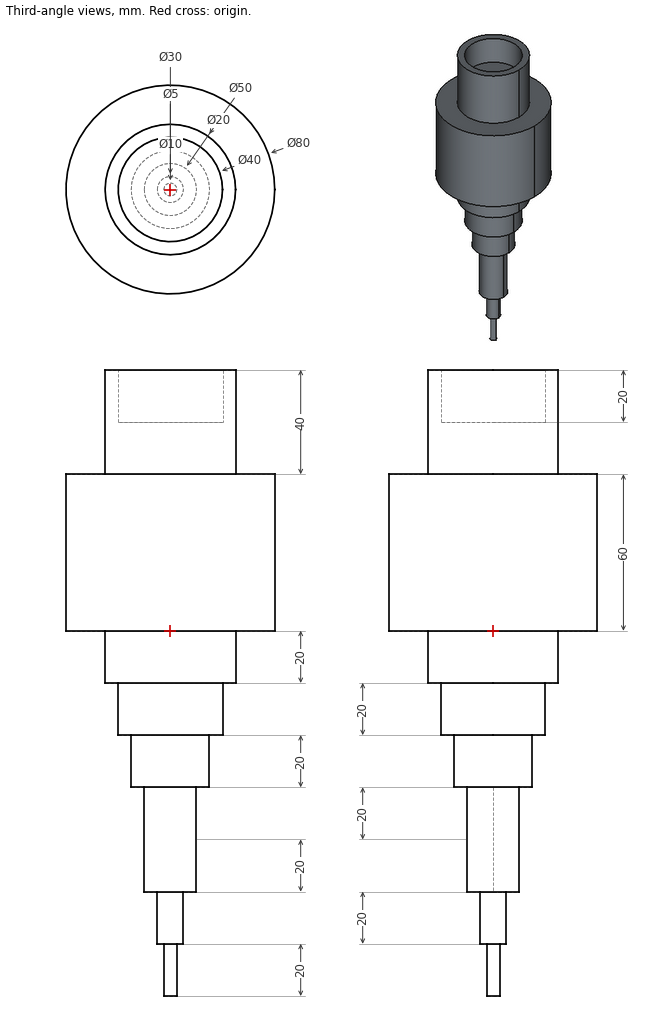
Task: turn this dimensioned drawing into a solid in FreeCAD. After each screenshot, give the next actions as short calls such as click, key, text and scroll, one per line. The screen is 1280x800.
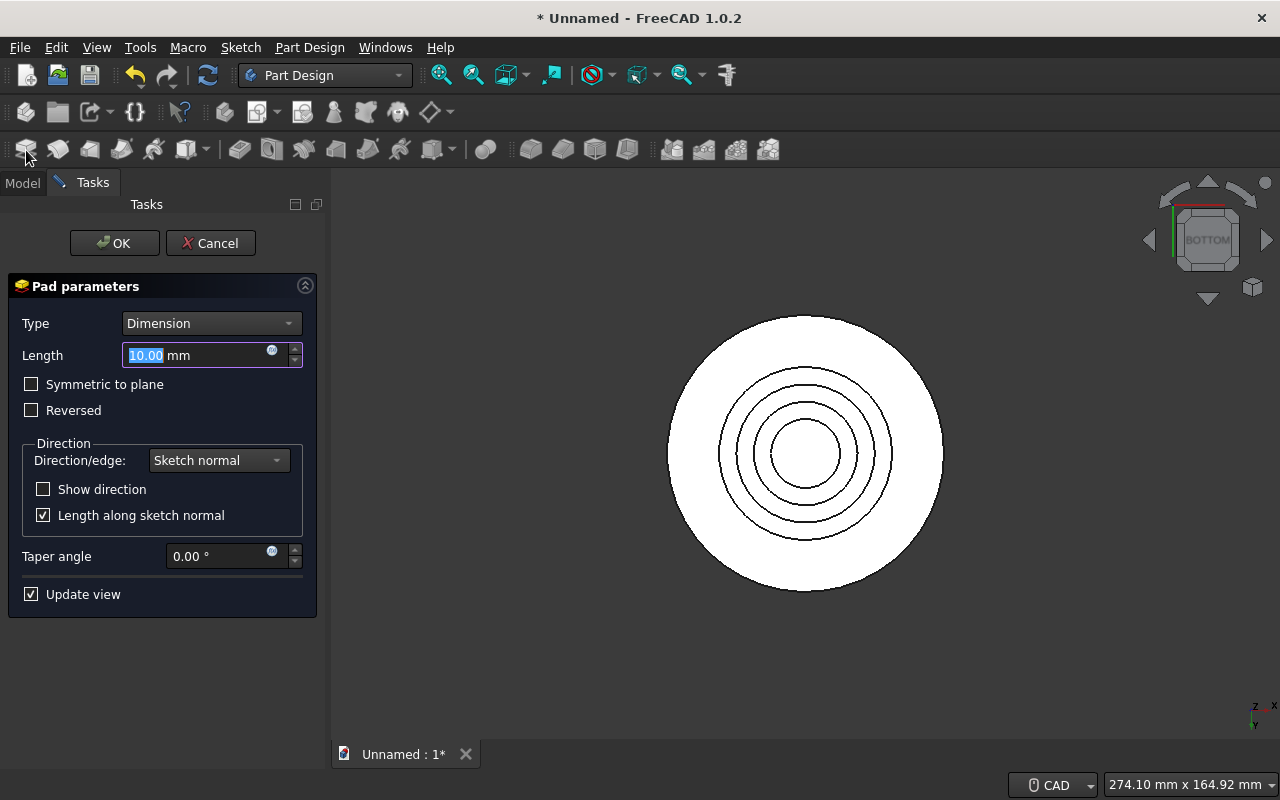
text(20)
key(Tab)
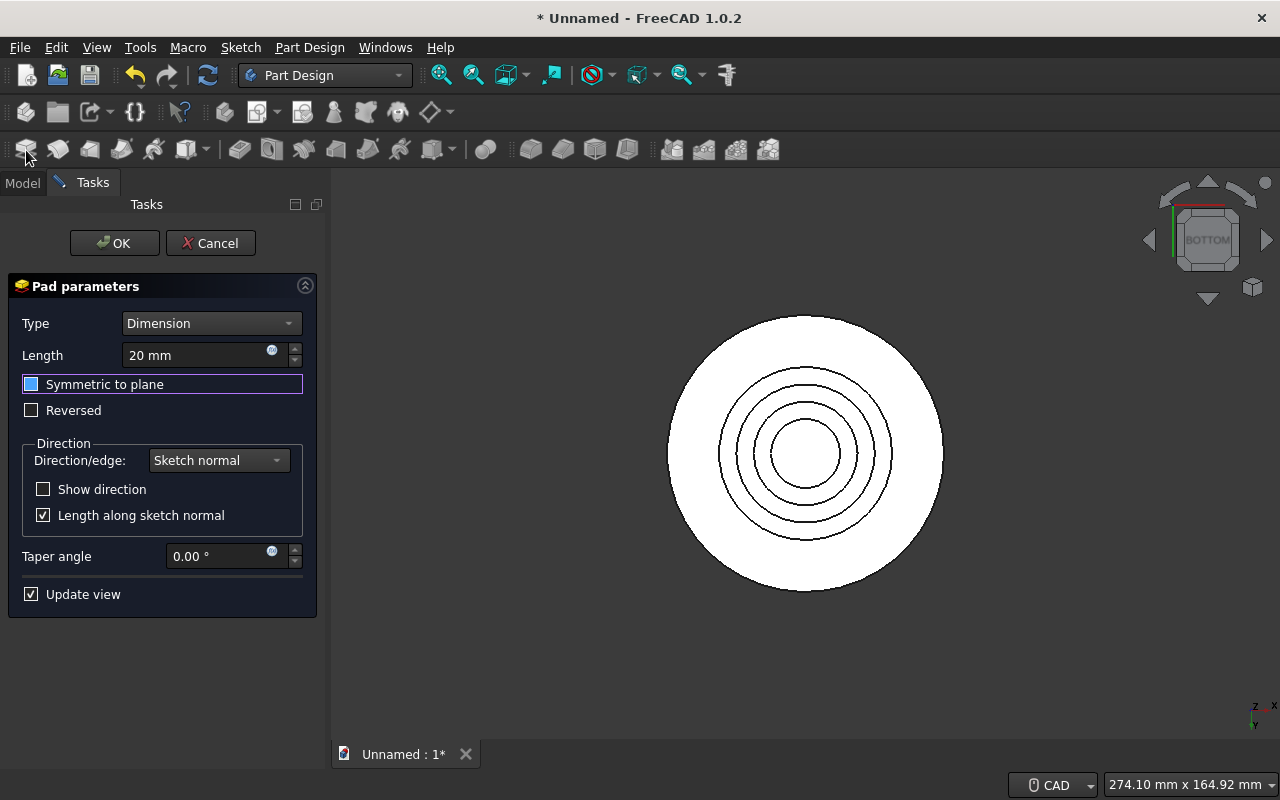
click(115, 243)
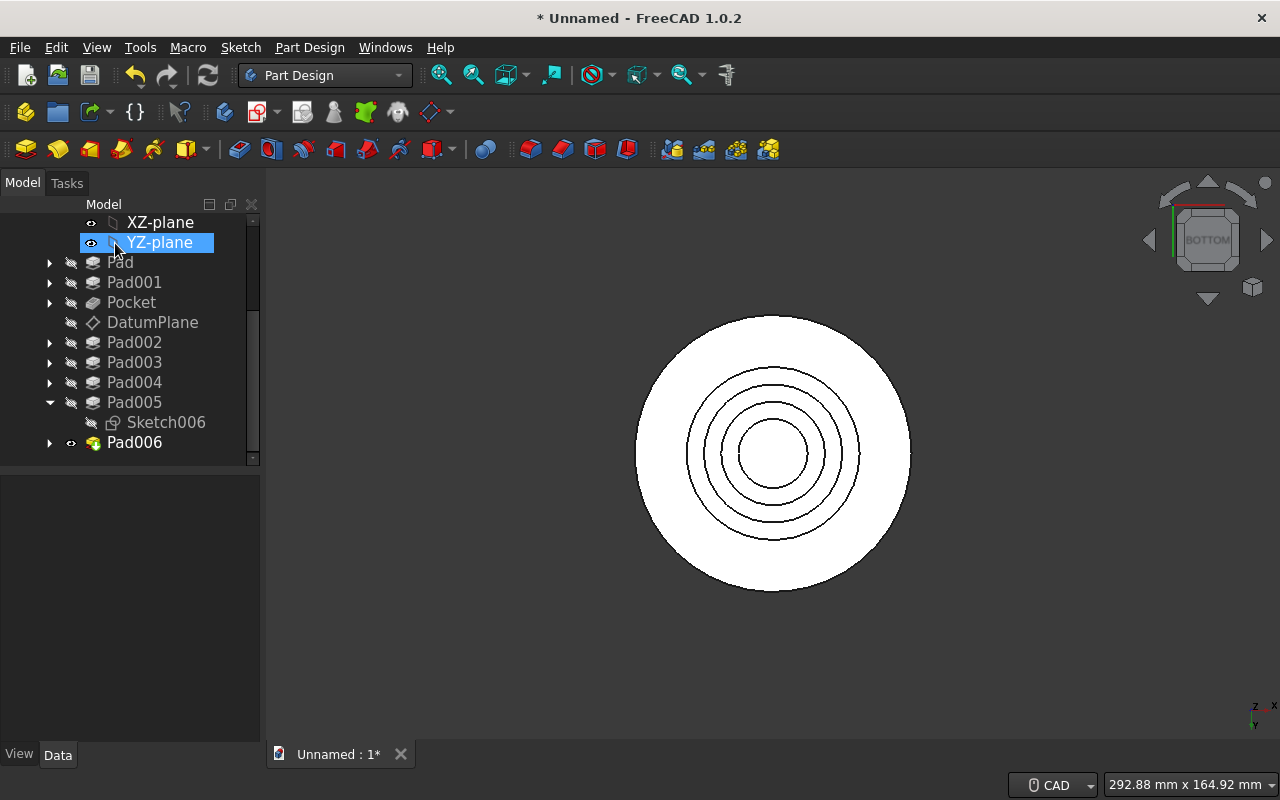
click(773, 452)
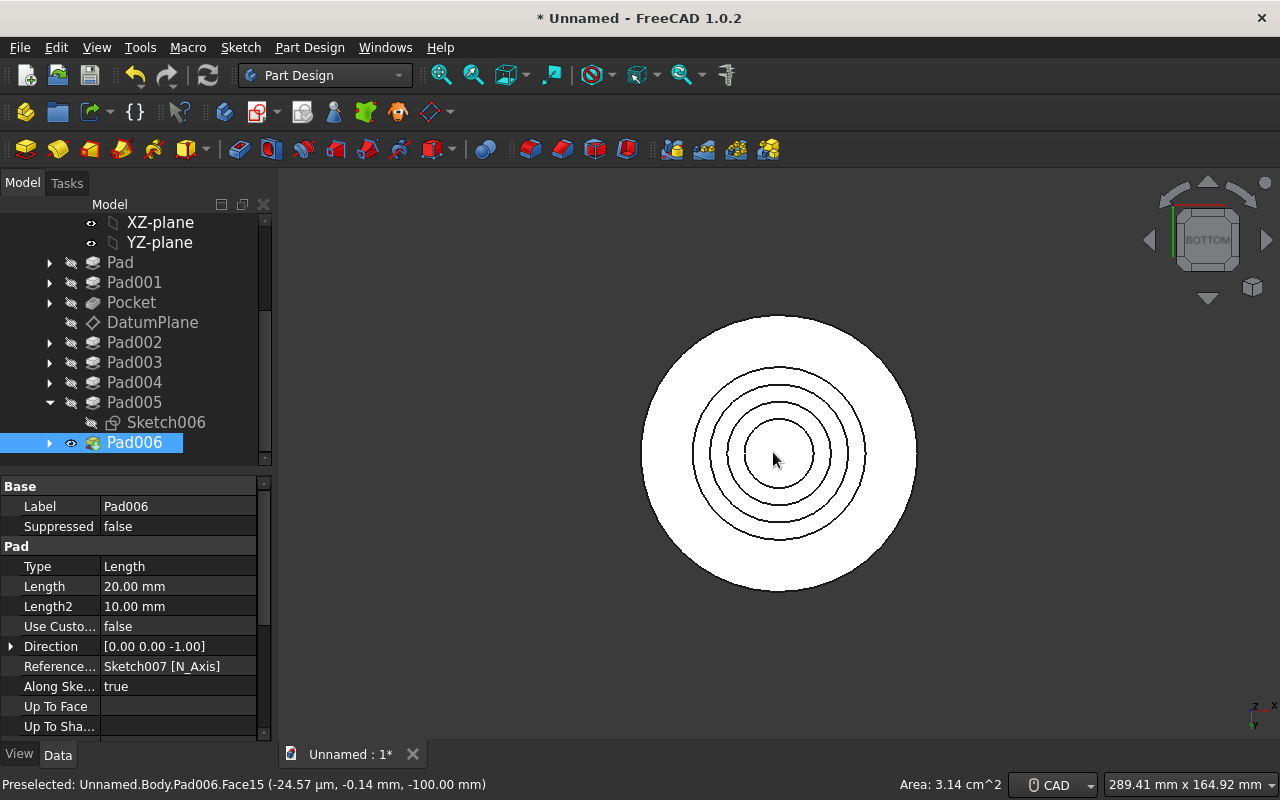
click(258, 112)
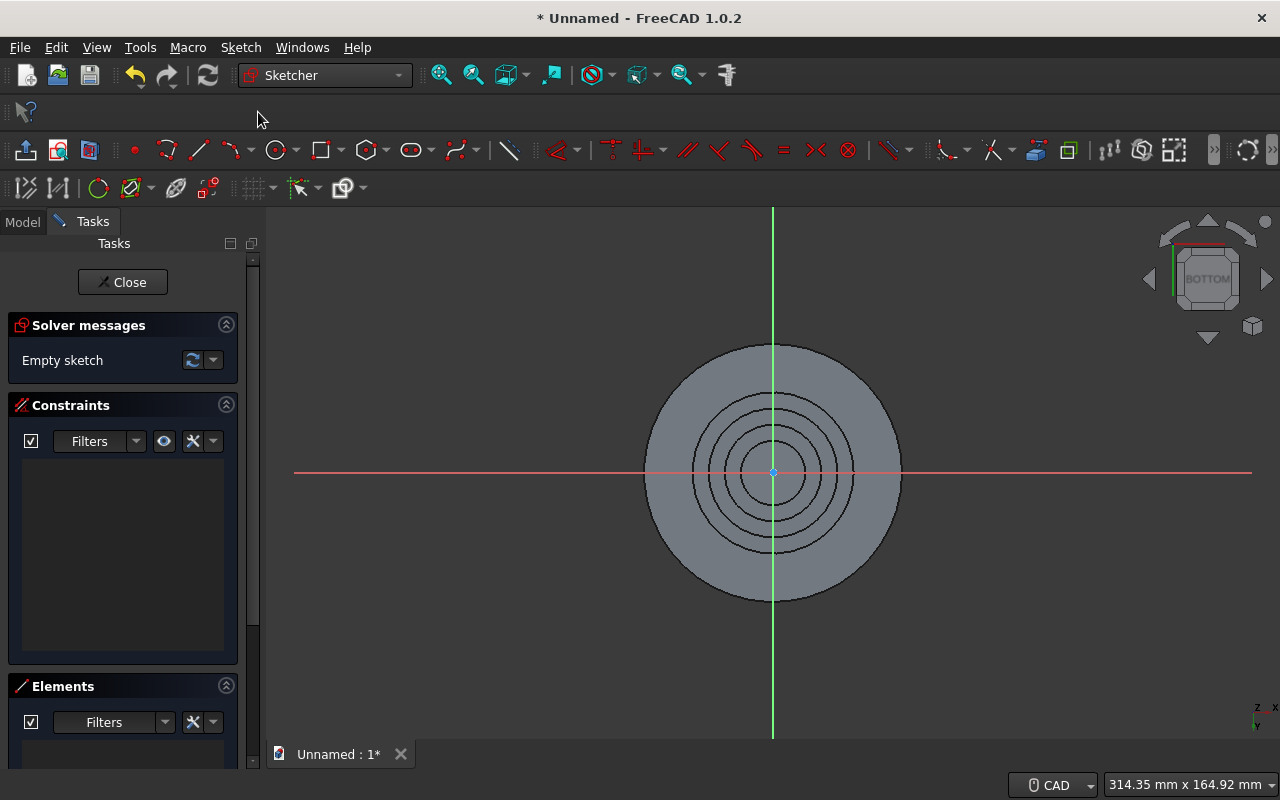
scroll(780, 473, up, 12)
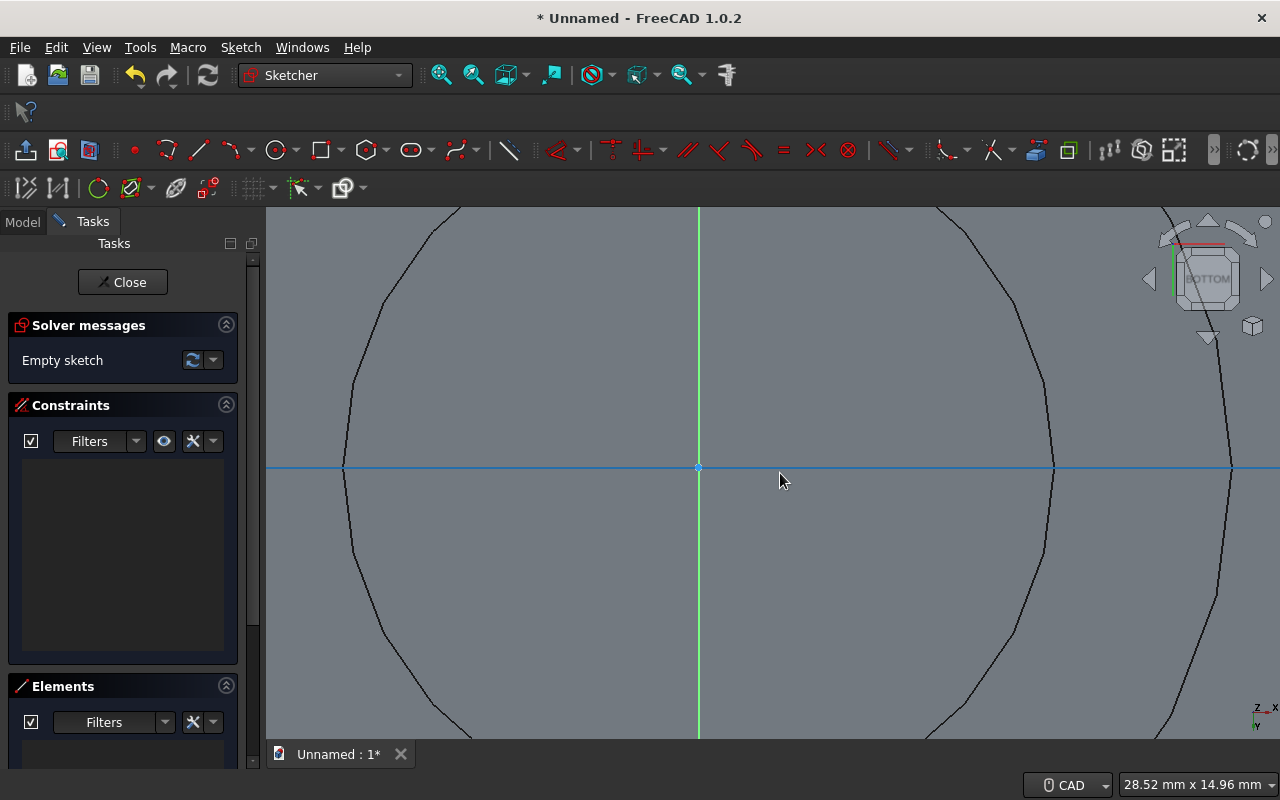
click(276, 150)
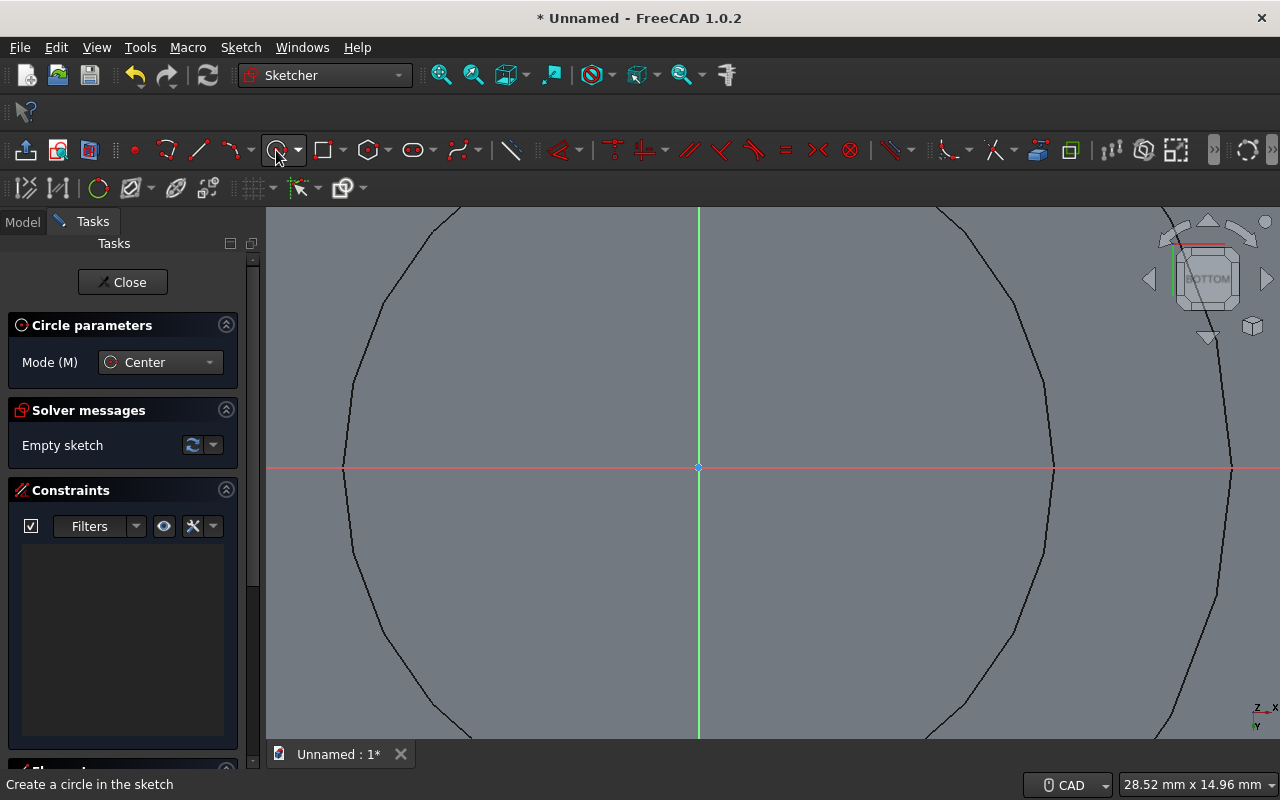
click(699, 468)
click(824, 342)
key(Escape)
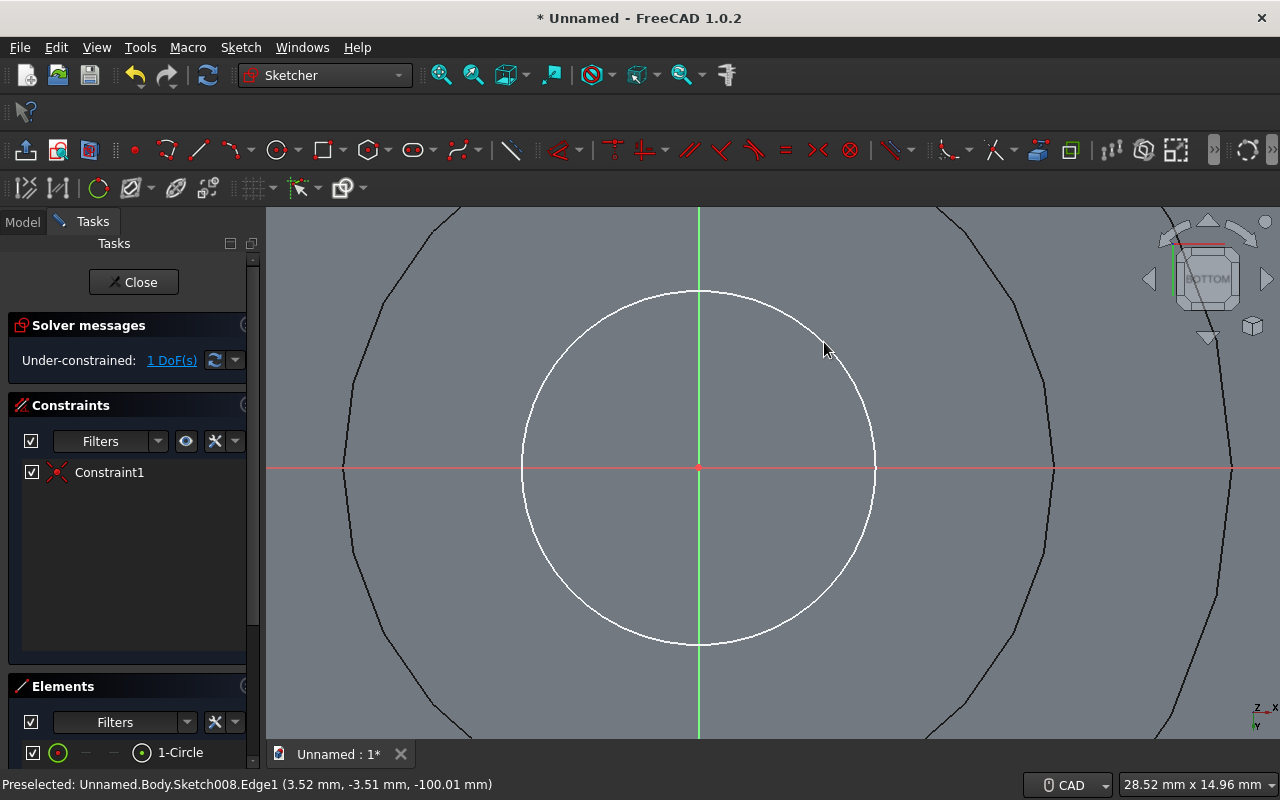
click(558, 150)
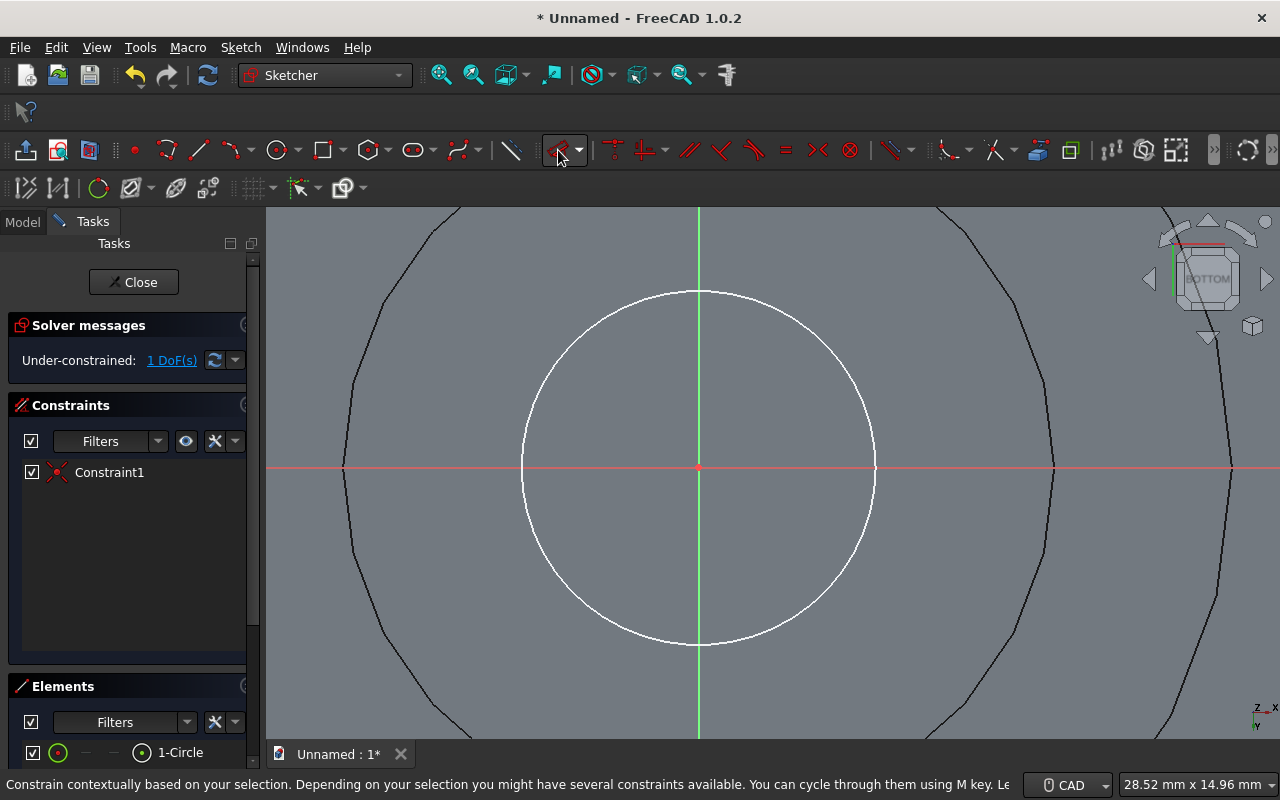
click(823, 342)
click(845, 319)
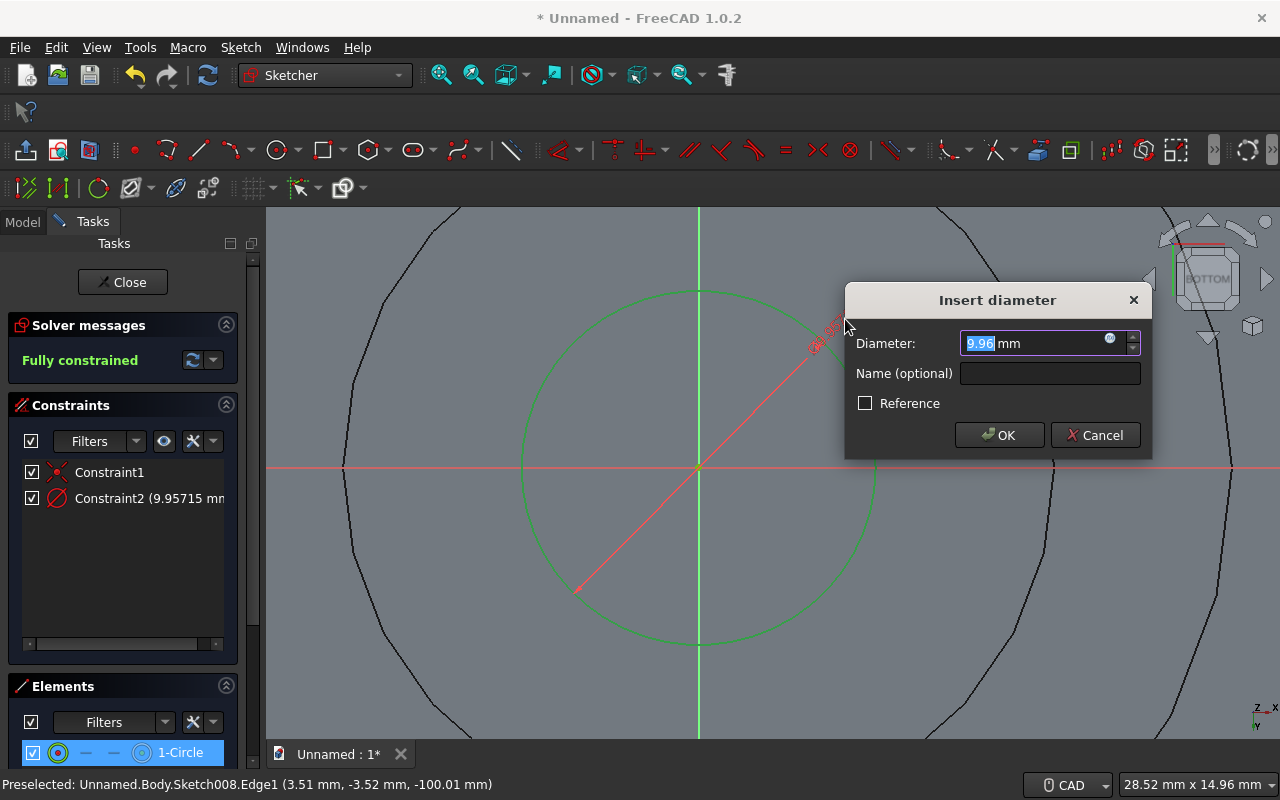
text(10)
key(Return)
key(Escape)